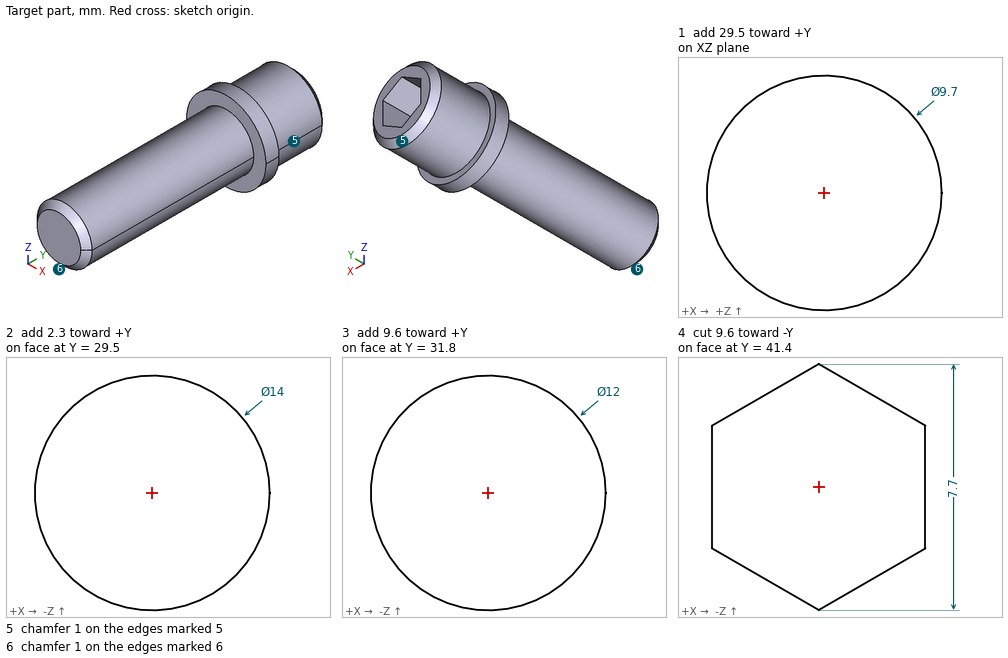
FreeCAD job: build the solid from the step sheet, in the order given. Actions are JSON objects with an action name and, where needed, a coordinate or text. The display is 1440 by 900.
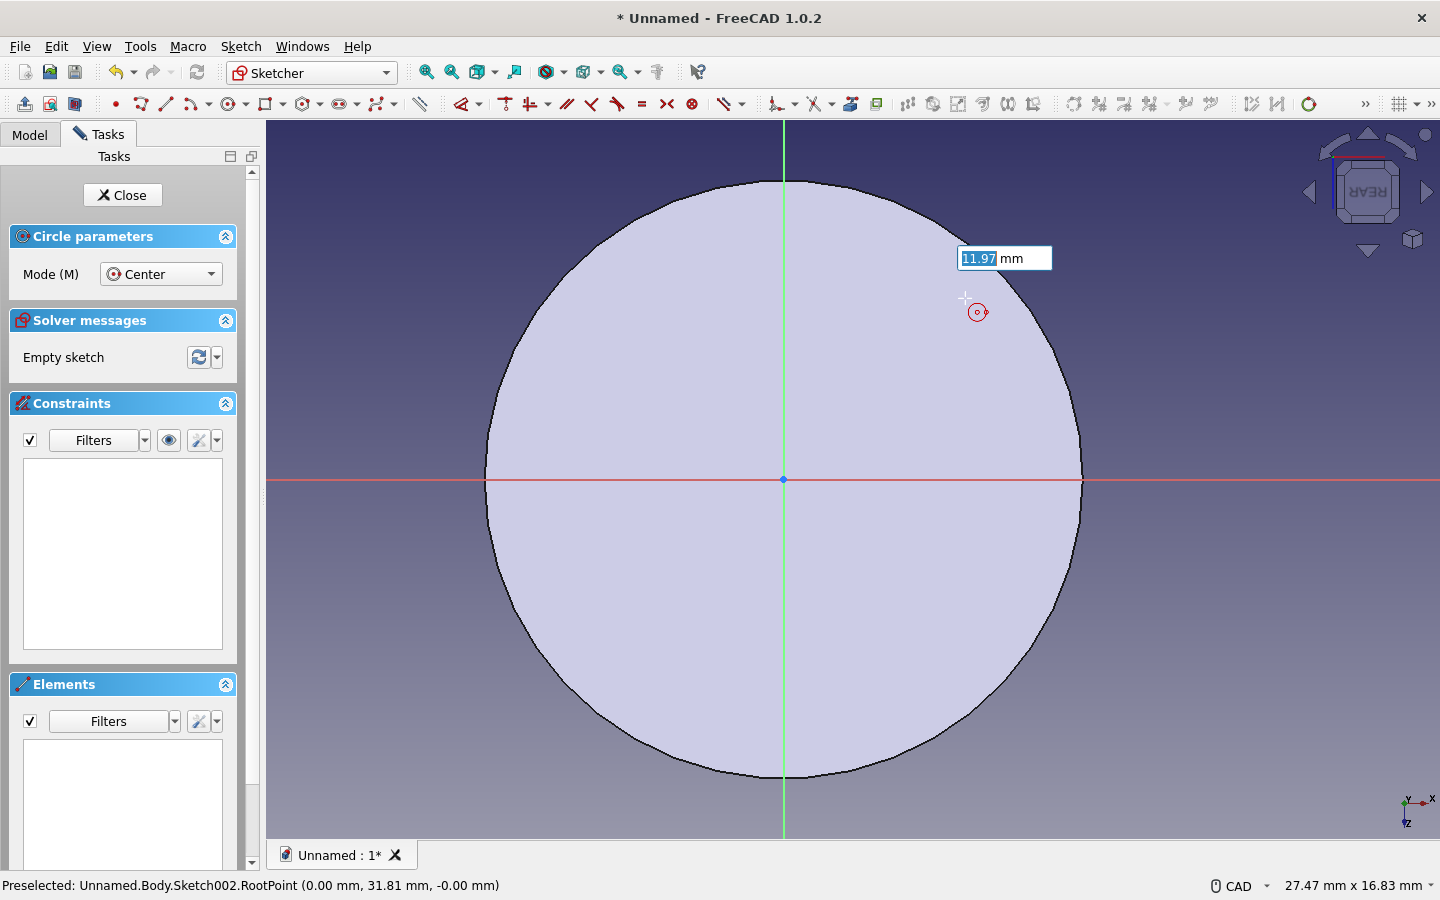
{"action": "type", "text": "12"}
{"action": "key", "text": "Return"}
{"action": "key", "text": "Escape"}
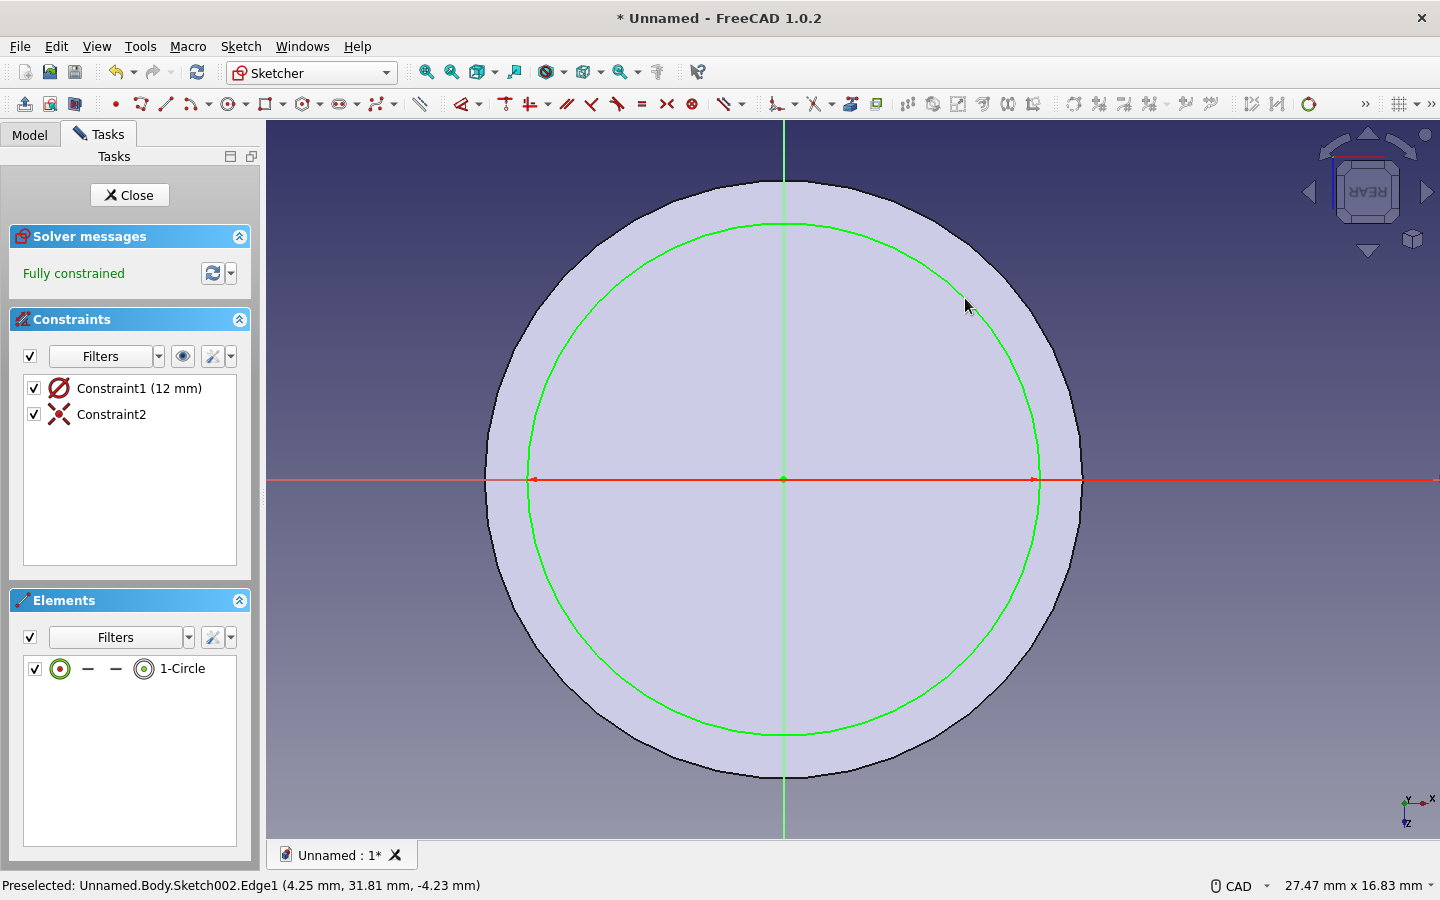
{"action": "left_click", "coordinate": [130, 195]}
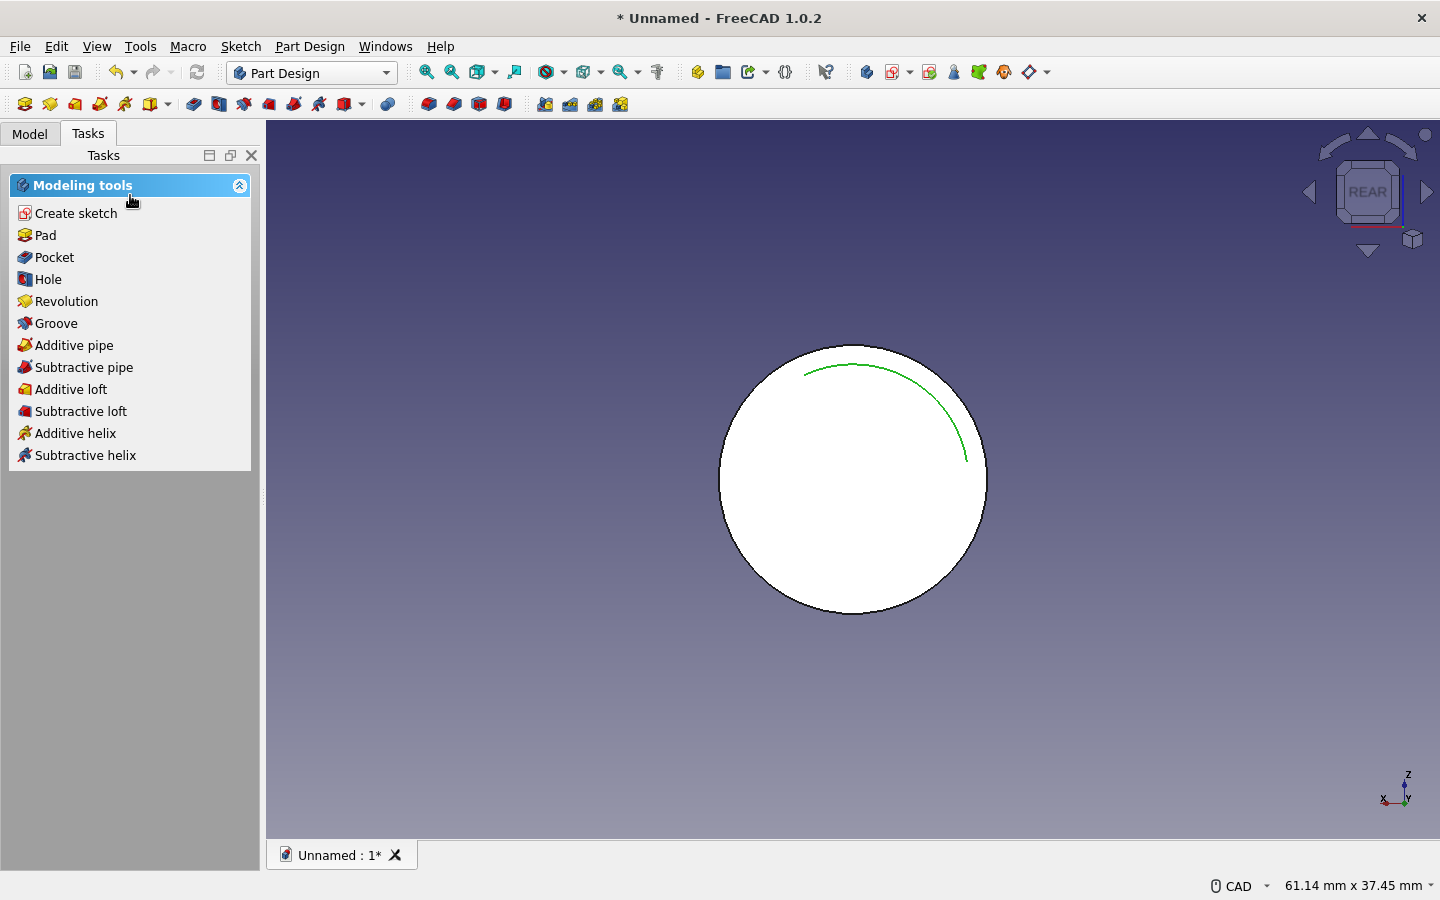
{"action": "left_click", "coordinate": [25, 104]}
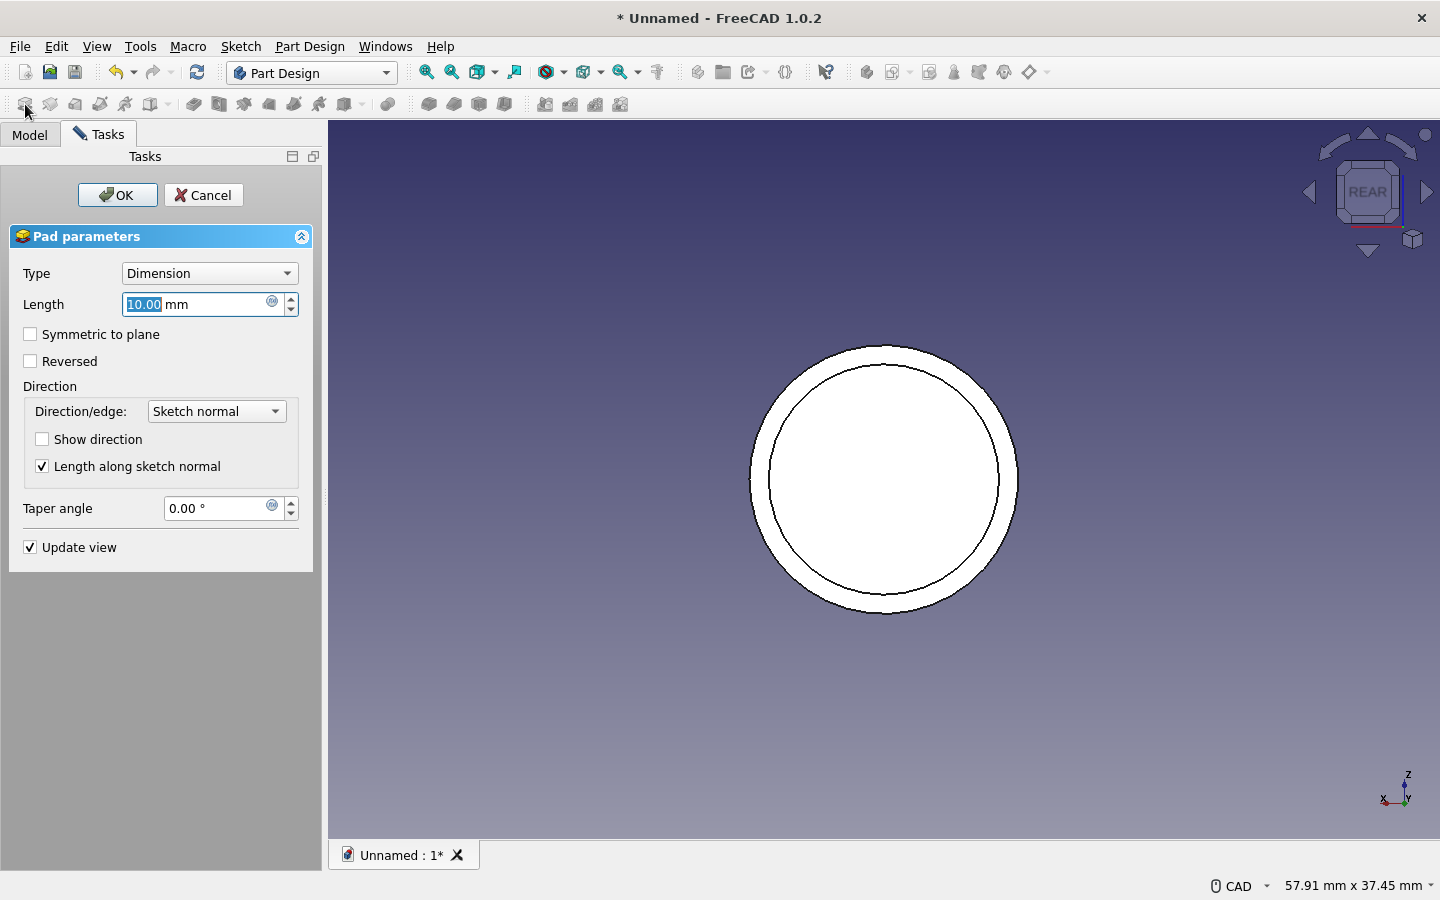
{"action": "type", "text": "9.6"}
{"action": "key", "text": "Tab"}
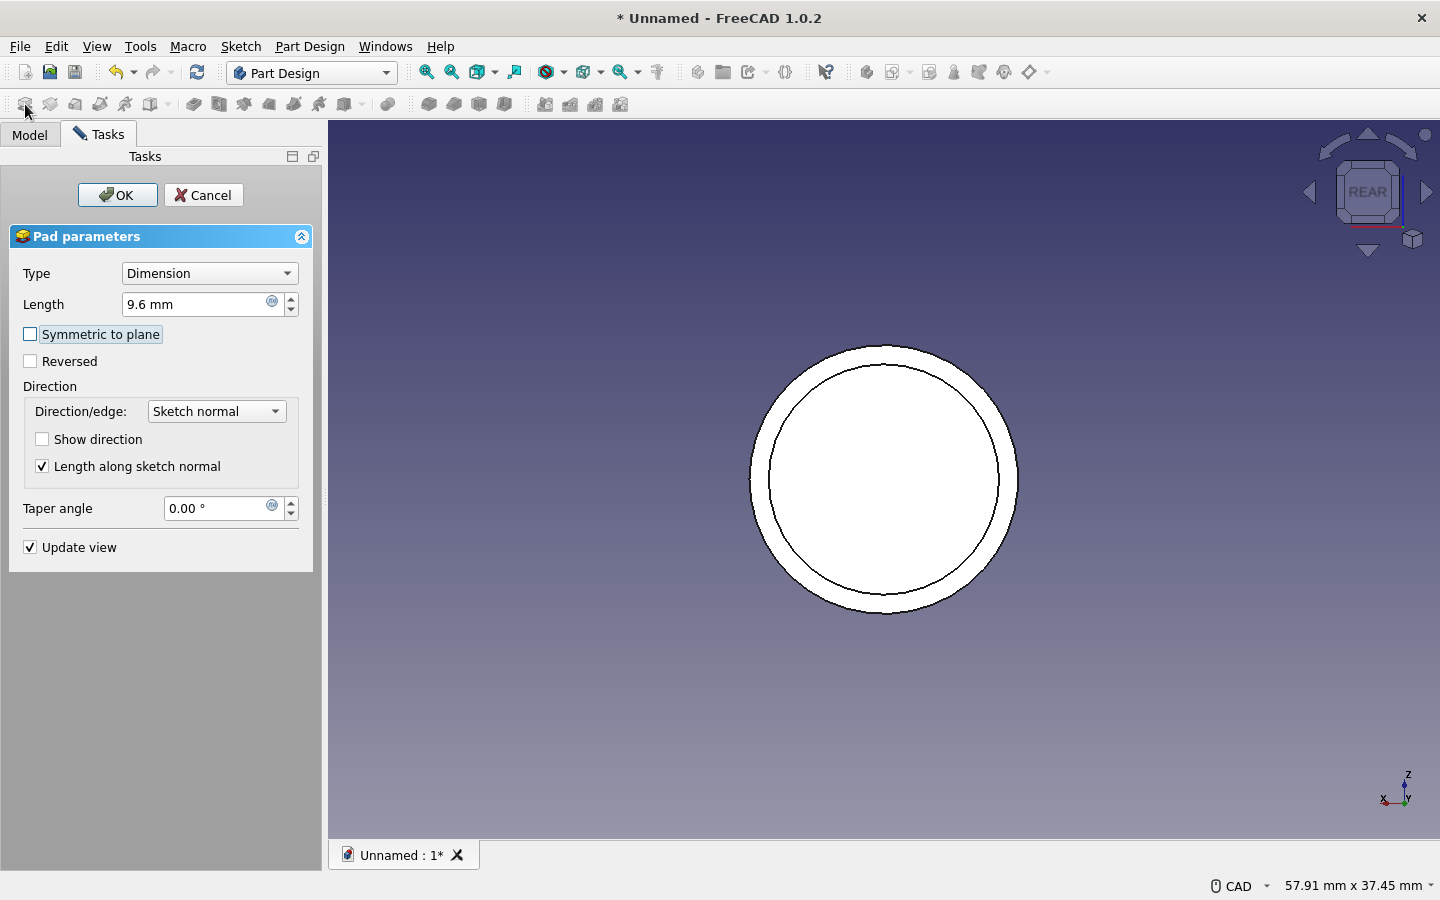
{"action": "left_click", "coordinate": [118, 195]}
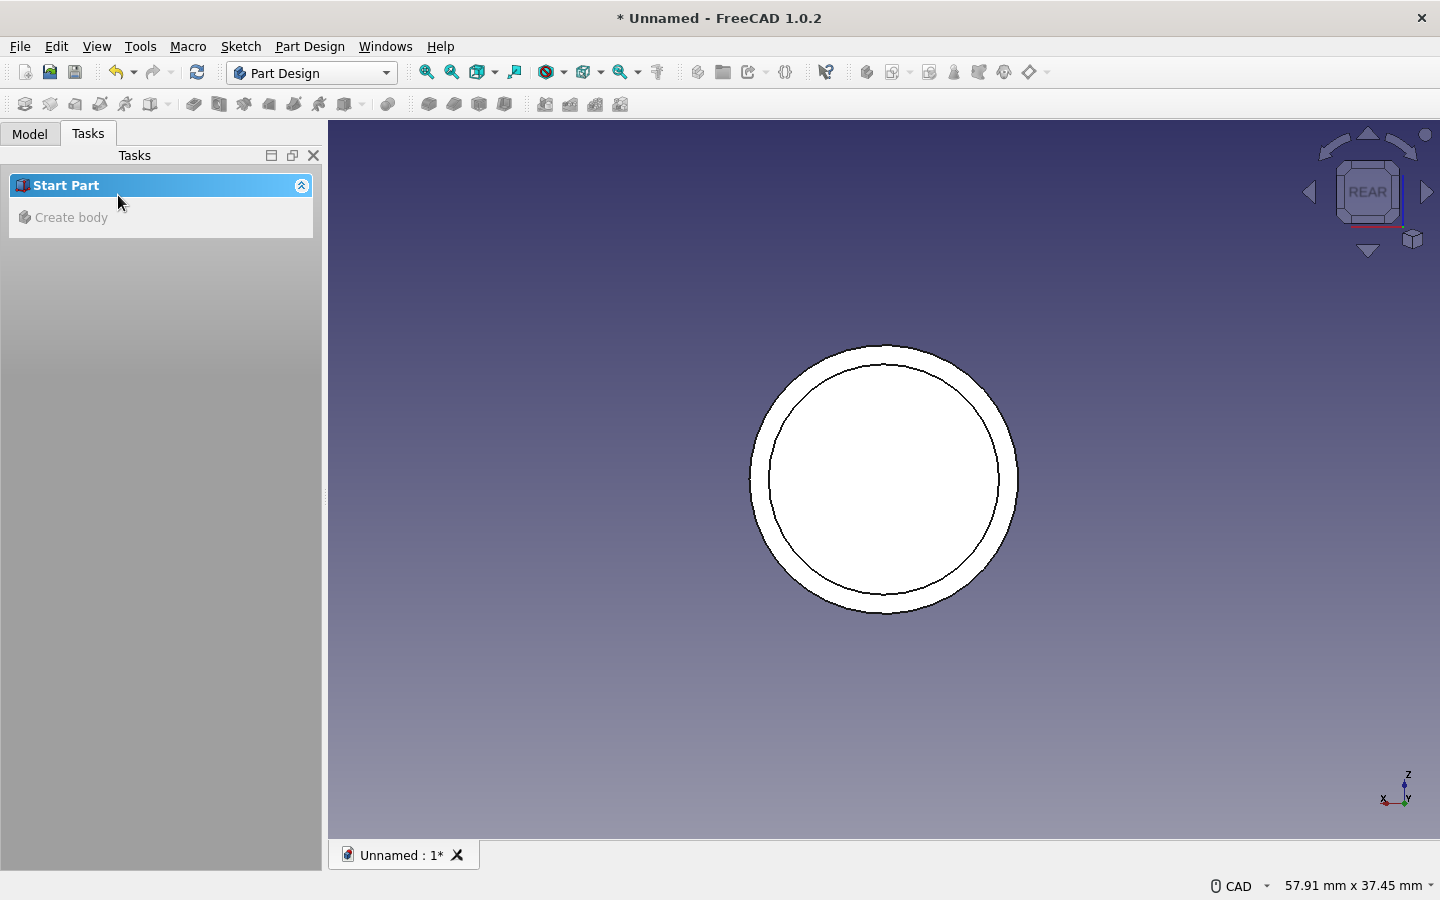
{"action": "left_click", "coordinate": [427, 72]}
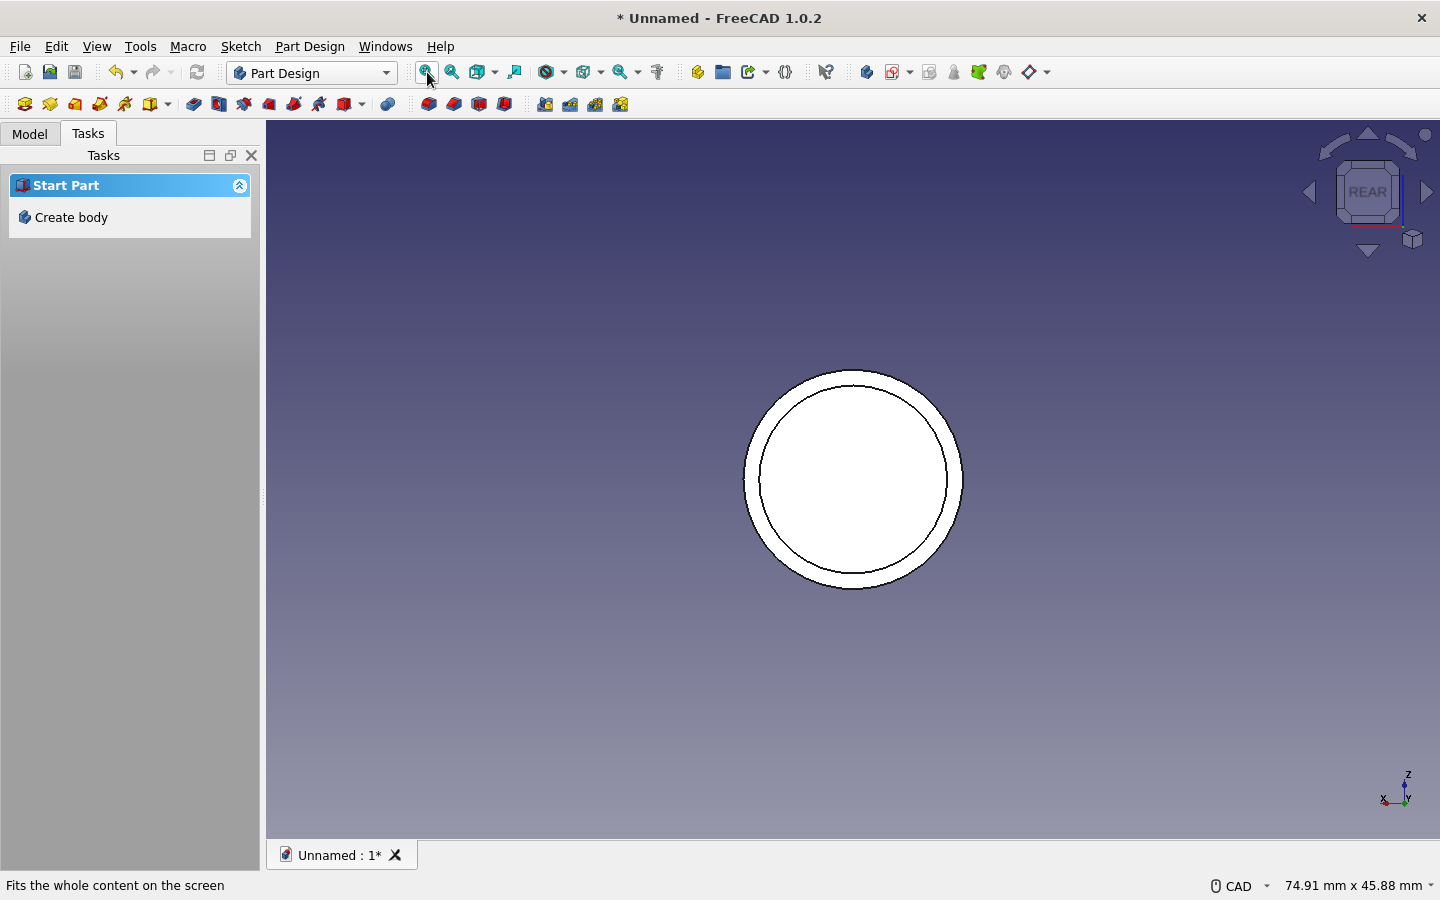
{"action": "left_click", "coordinate": [853, 478]}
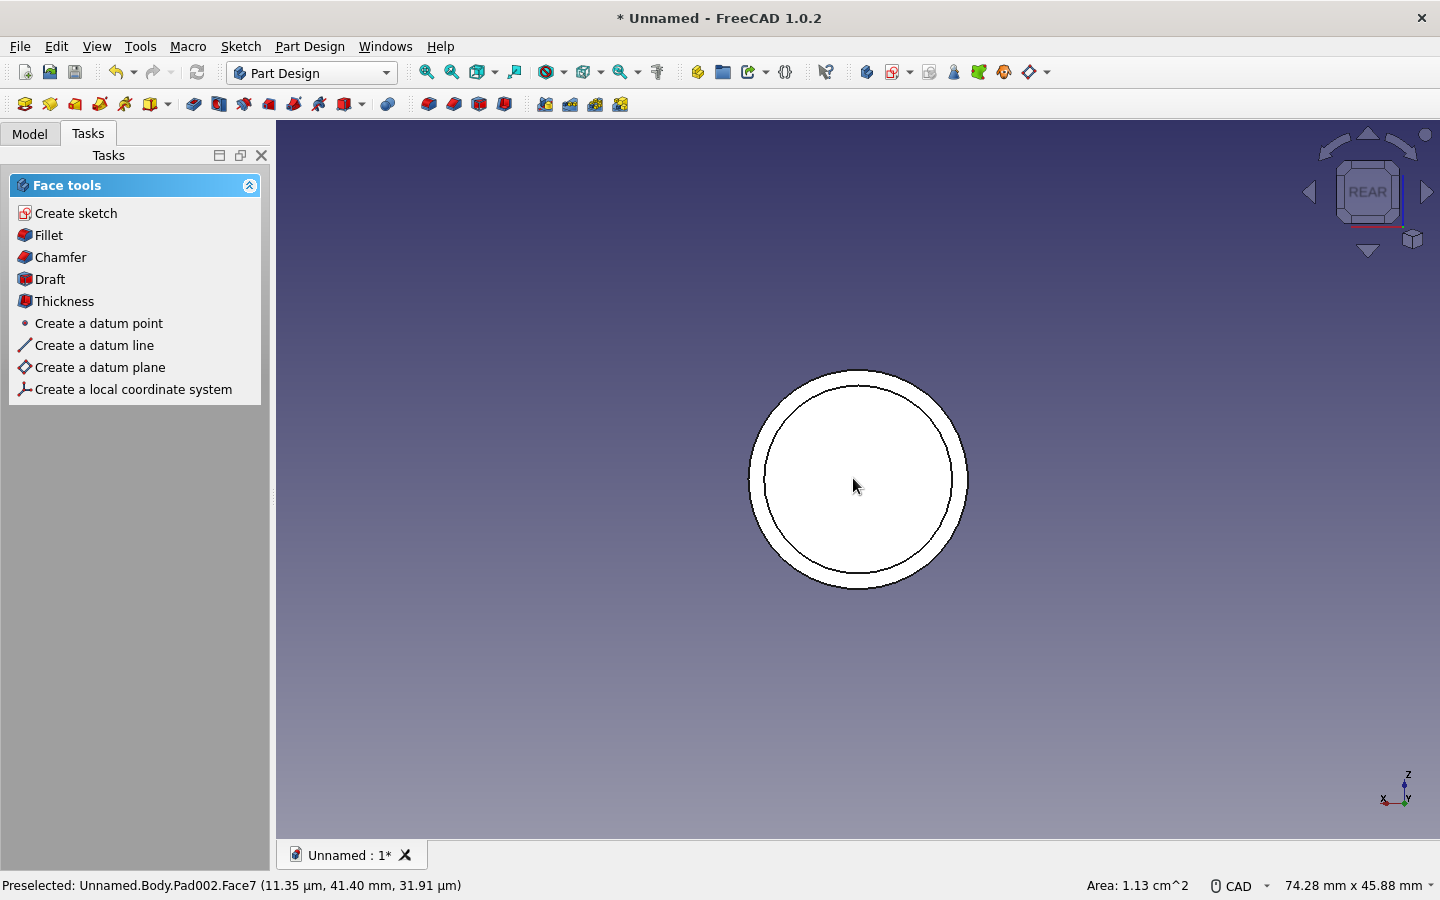
{"action": "left_click", "coordinate": [892, 72]}